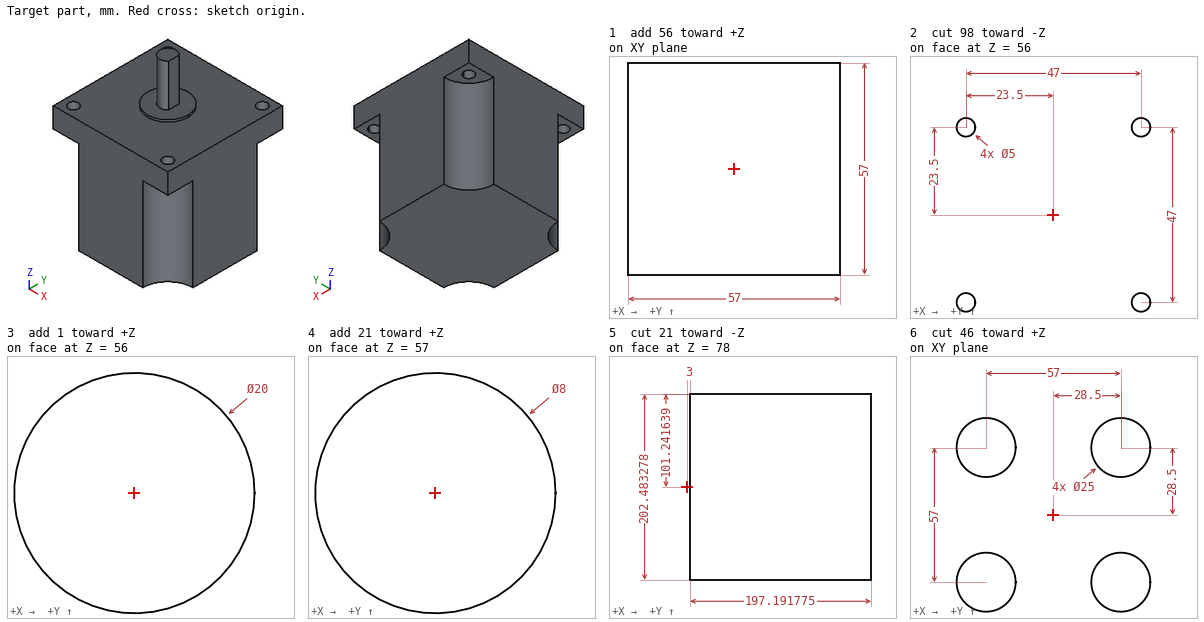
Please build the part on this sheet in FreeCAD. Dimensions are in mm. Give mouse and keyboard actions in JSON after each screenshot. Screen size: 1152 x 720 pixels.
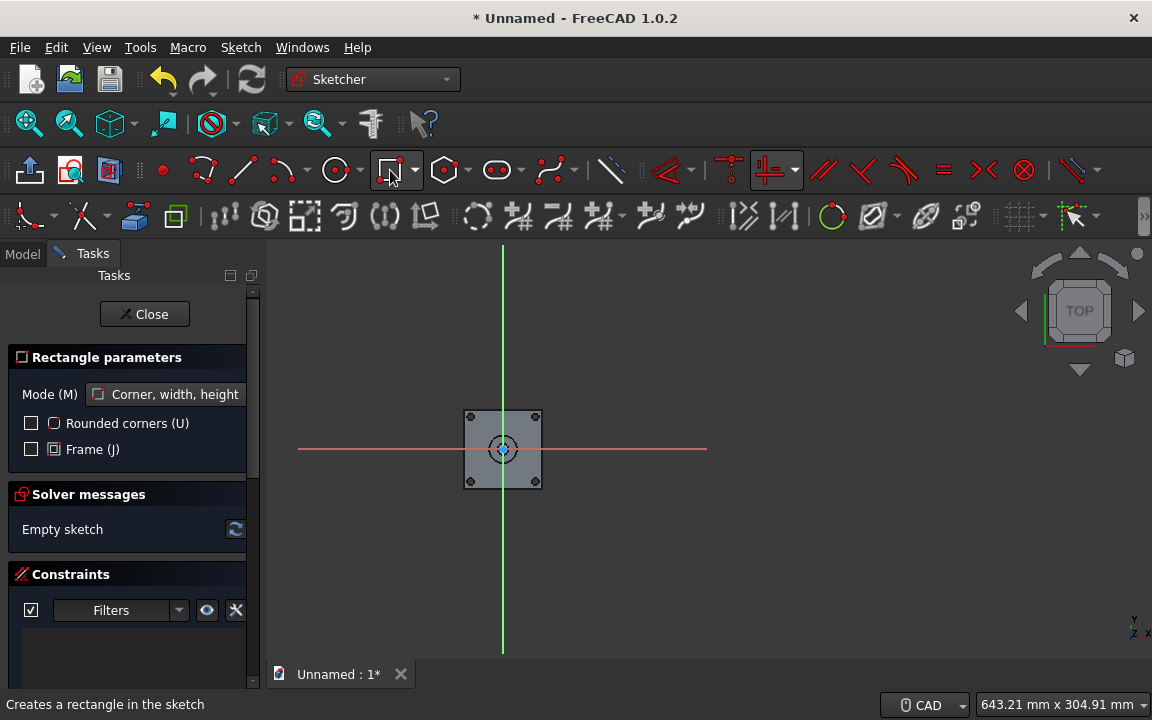
{"action": "scroll", "coordinate": [507, 310], "scroll_direction": "up", "scroll_amount": 7}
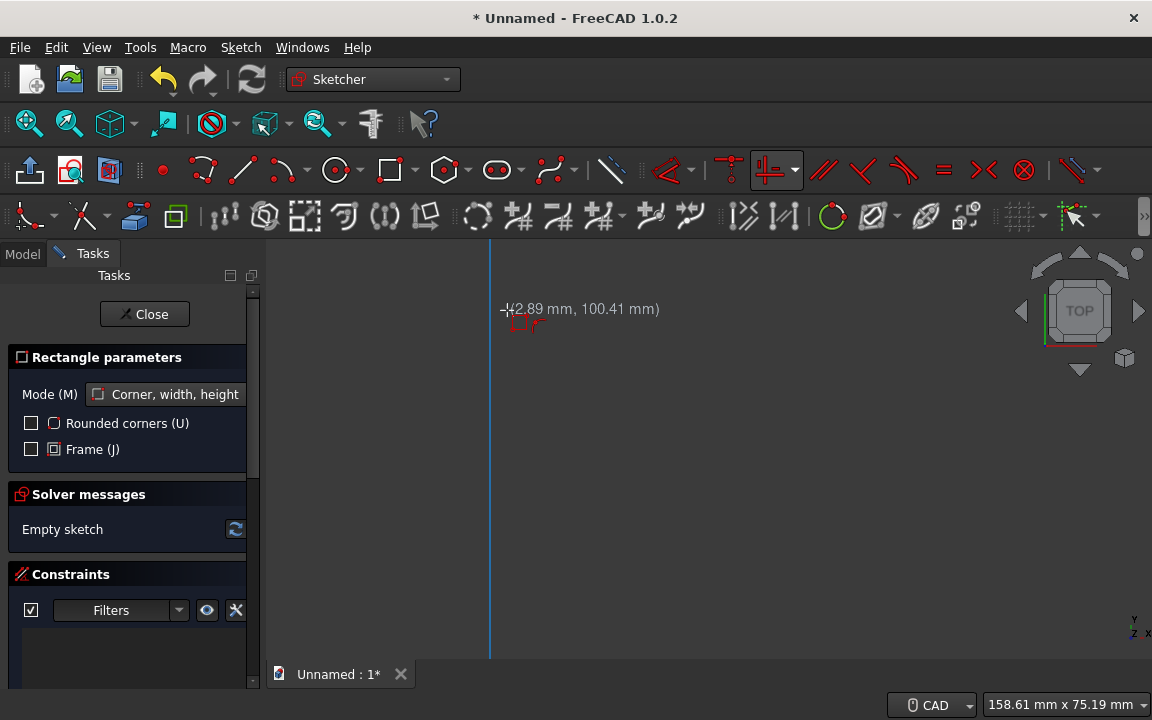
{"action": "left_click", "coordinate": [507, 309]}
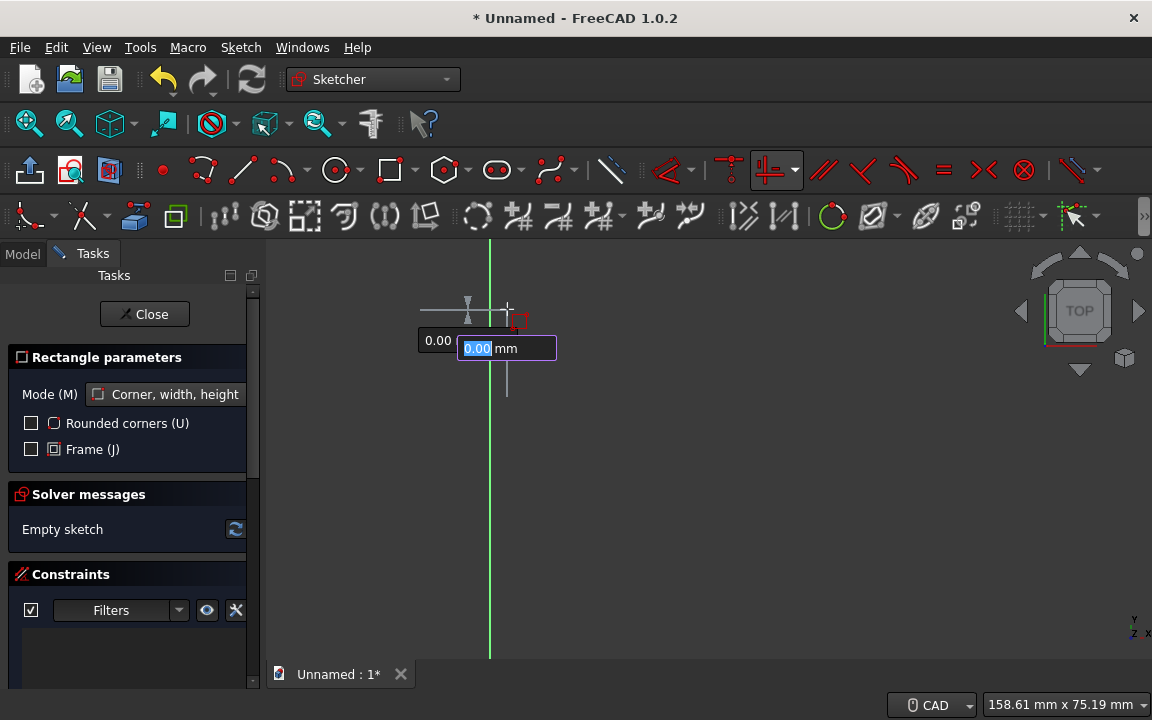
{"action": "scroll", "coordinate": [507, 310], "scroll_direction": "down", "scroll_amount": 7}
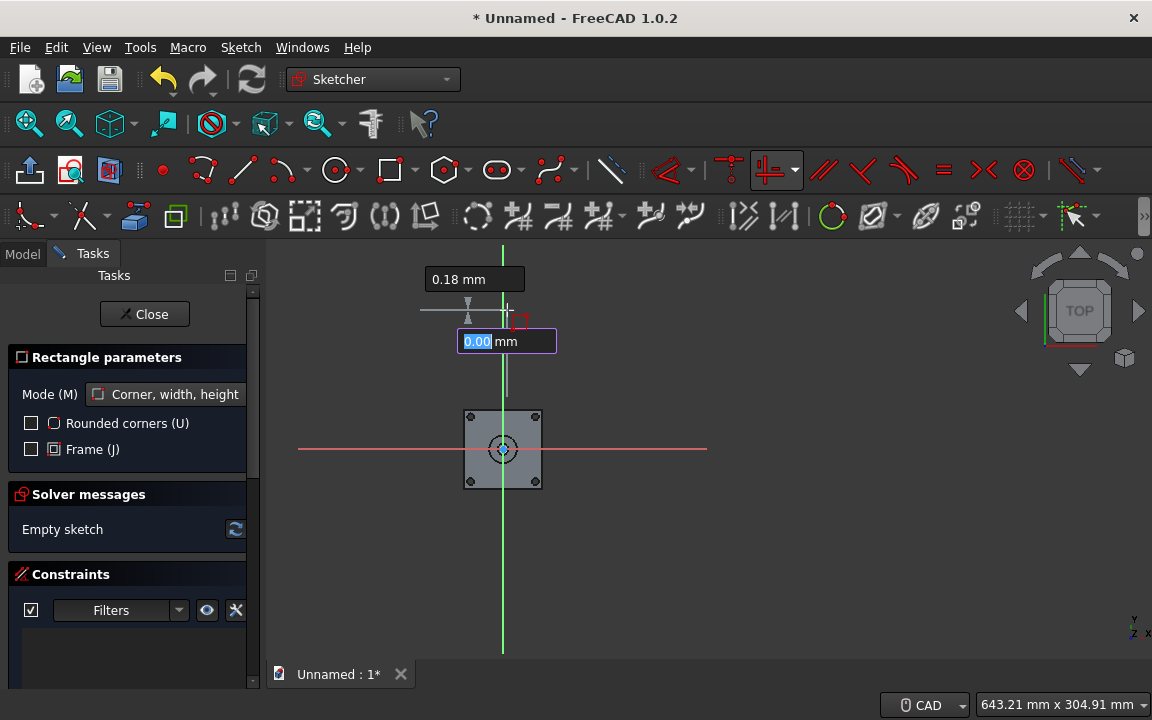
{"action": "left_click", "coordinate": [779, 589]}
{"action": "key", "text": "Escape"}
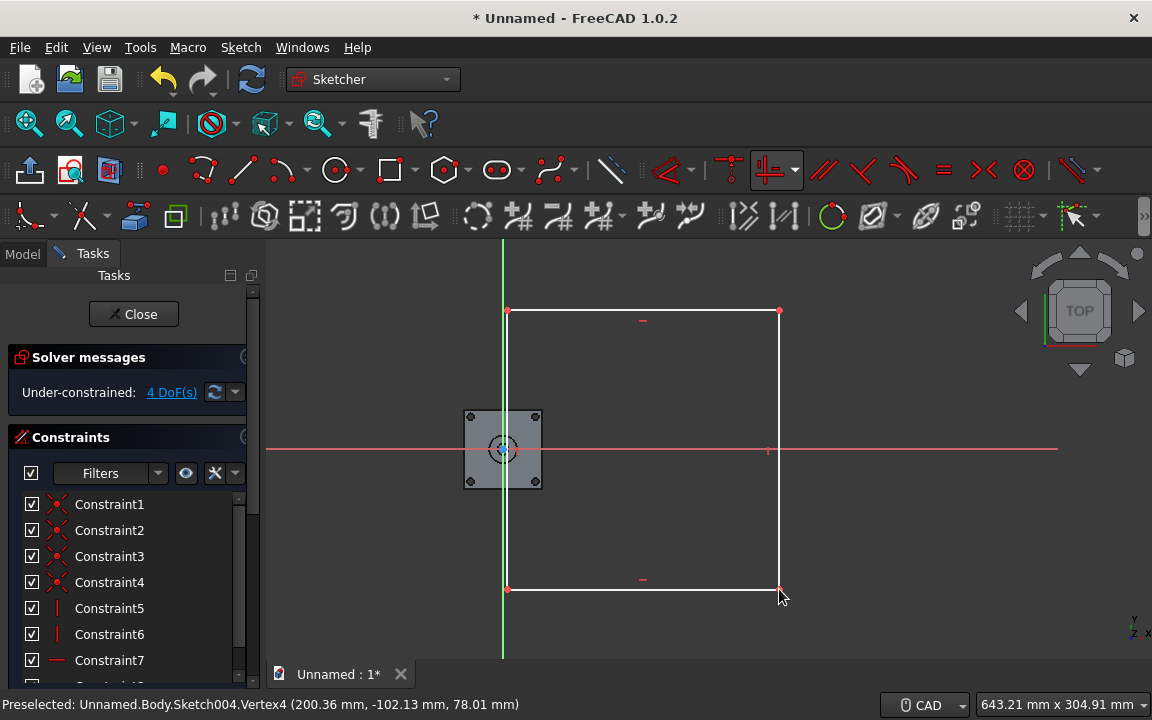
{"action": "left_click", "coordinate": [666, 170]}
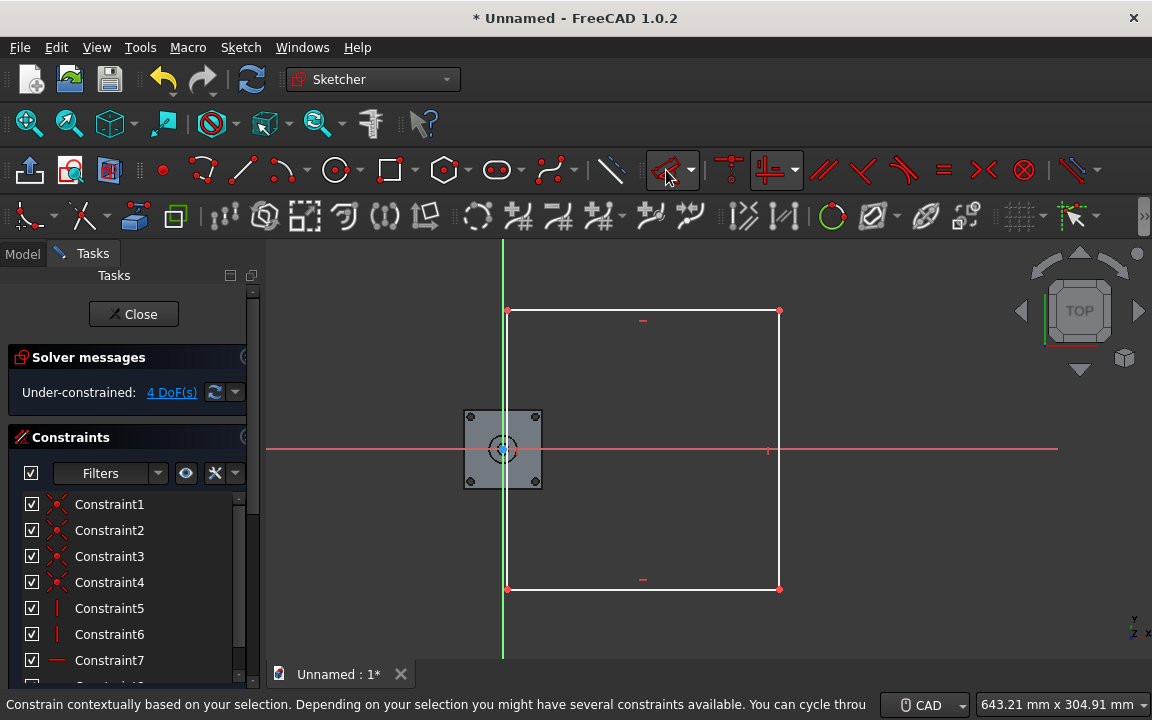
{"action": "scroll", "coordinate": [507, 310], "scroll_direction": "up", "scroll_amount": 12}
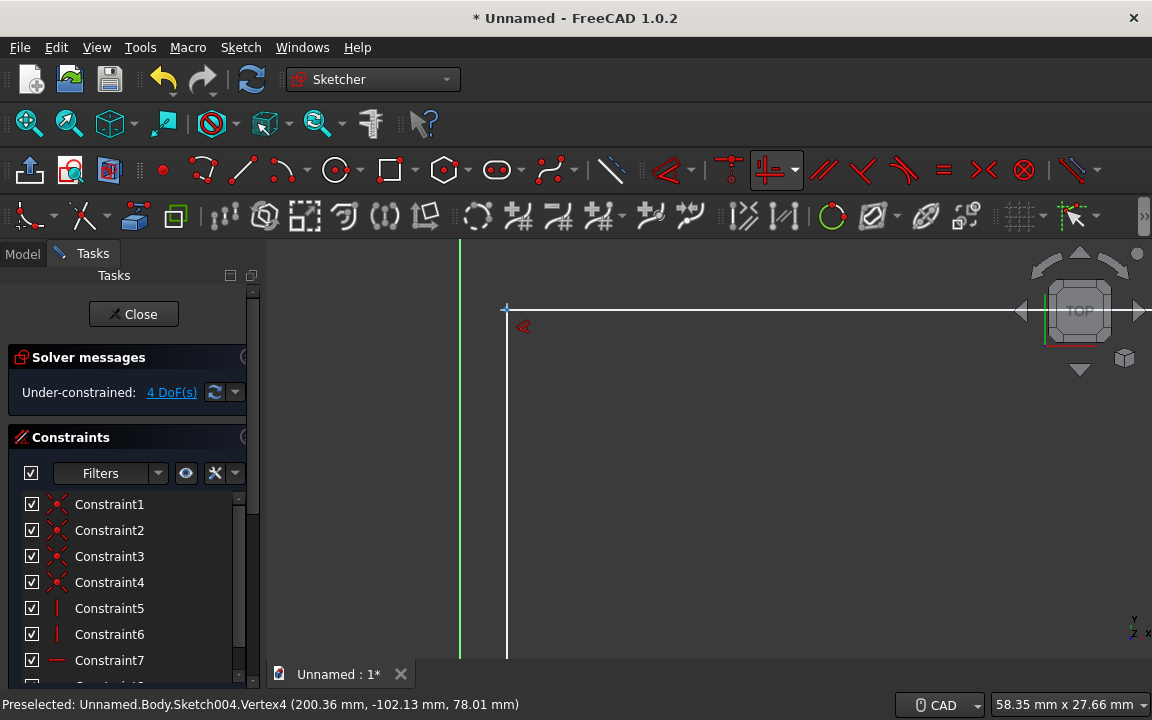
{"action": "left_click", "coordinate": [507, 310]}
{"action": "left_click", "coordinate": [483, 276]}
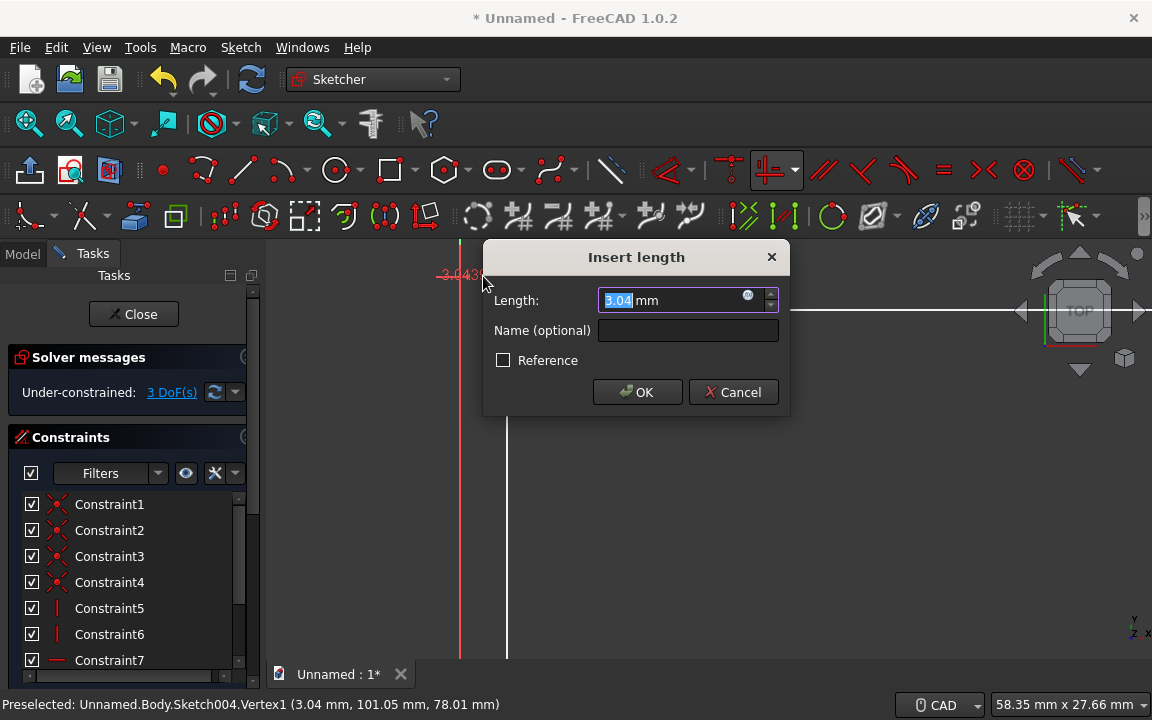
{"action": "type", "text": "3"}
{"action": "key", "text": "Return"}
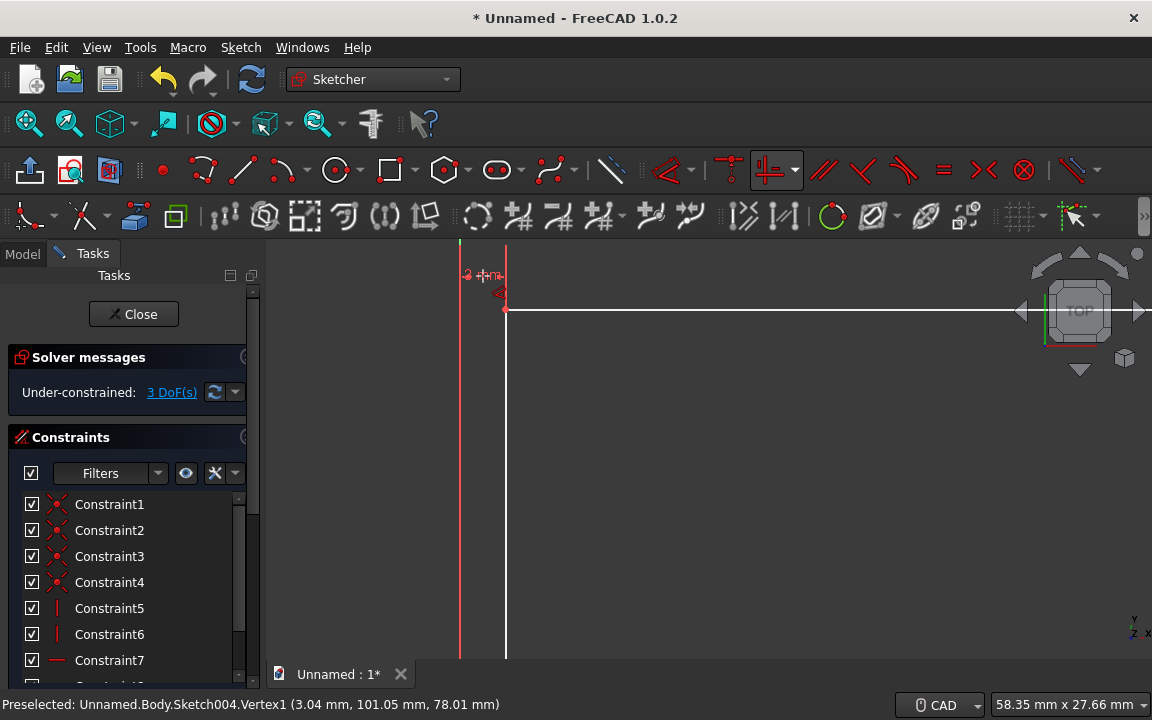
{"action": "scroll", "coordinate": [507, 310], "scroll_direction": "down", "scroll_amount": 12}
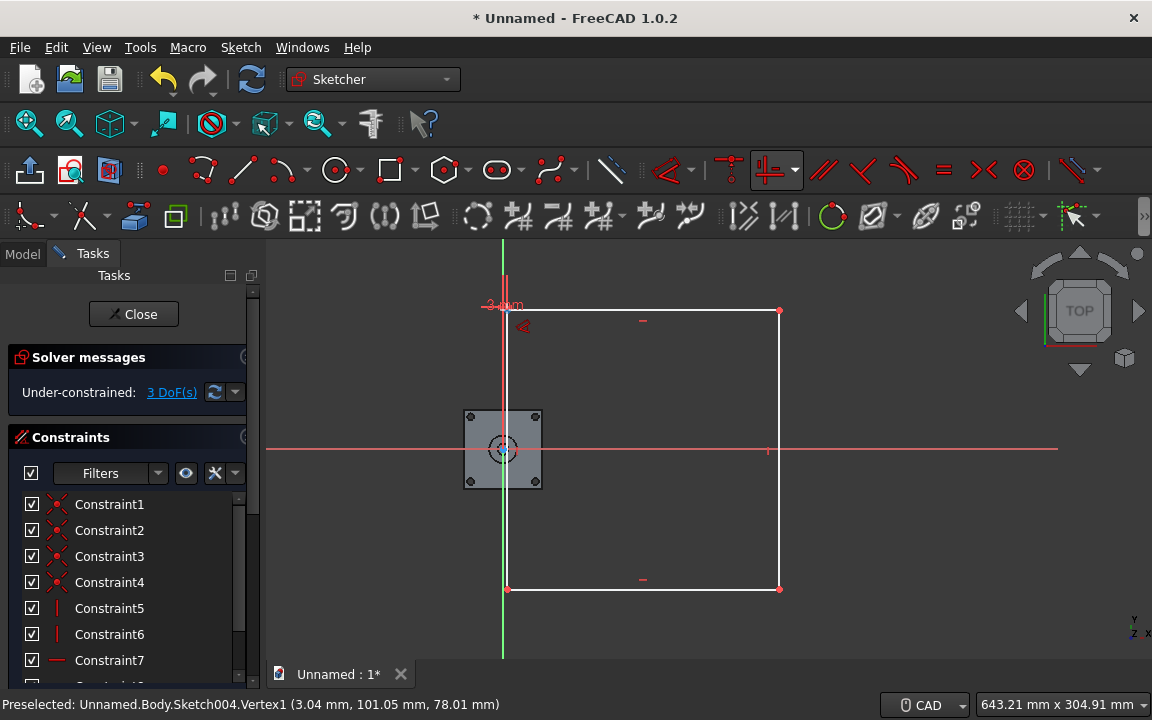
{"action": "scroll", "coordinate": [507, 394], "scroll_direction": "up", "scroll_amount": 7}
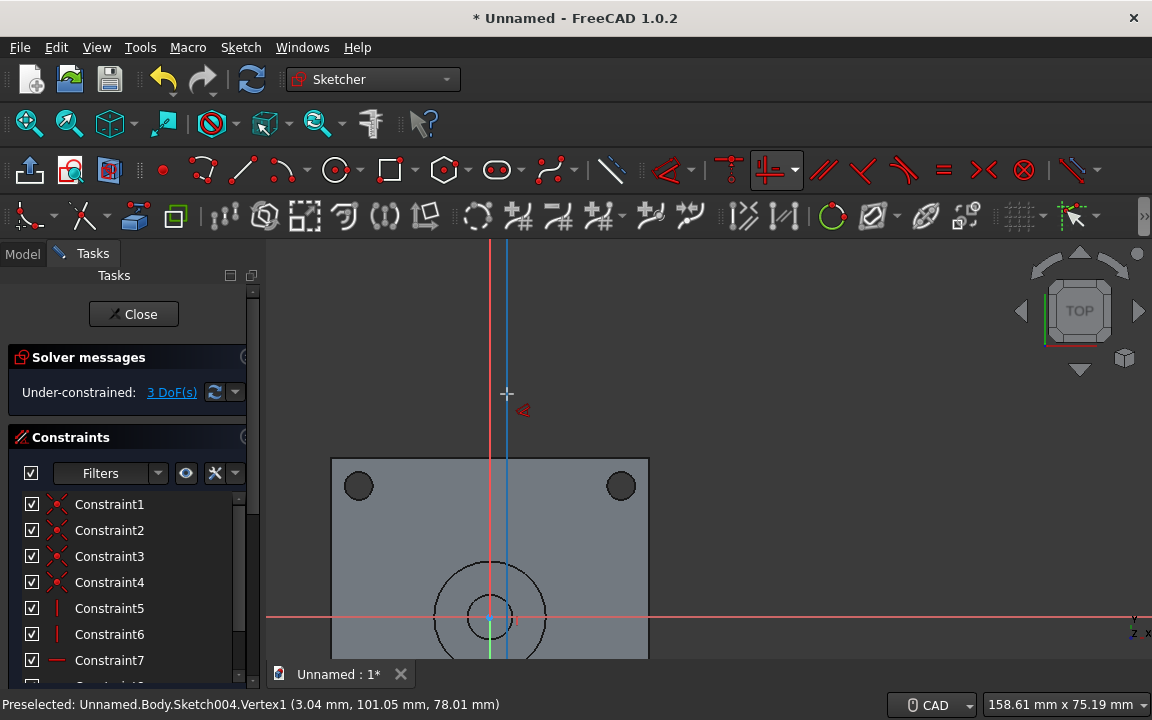
{"action": "left_click", "coordinate": [507, 393]}
{"action": "left_click", "coordinate": [473, 449]}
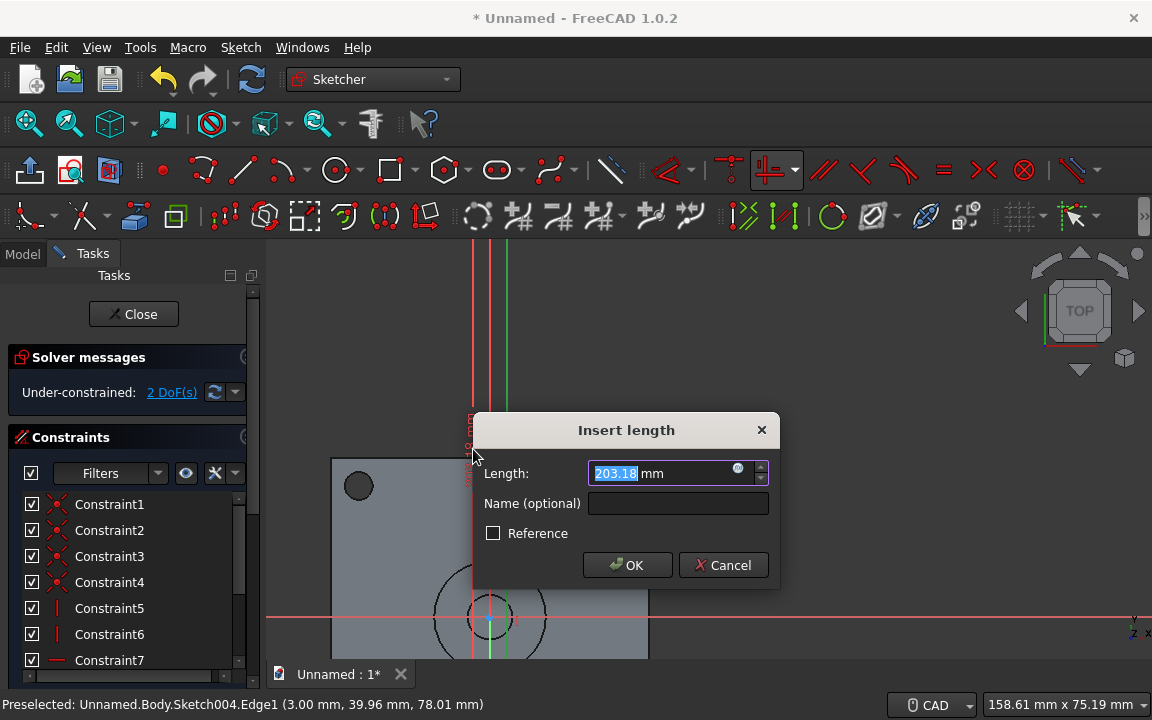
{"action": "type", "text": "202.483278"}
{"action": "key", "text": "Return"}